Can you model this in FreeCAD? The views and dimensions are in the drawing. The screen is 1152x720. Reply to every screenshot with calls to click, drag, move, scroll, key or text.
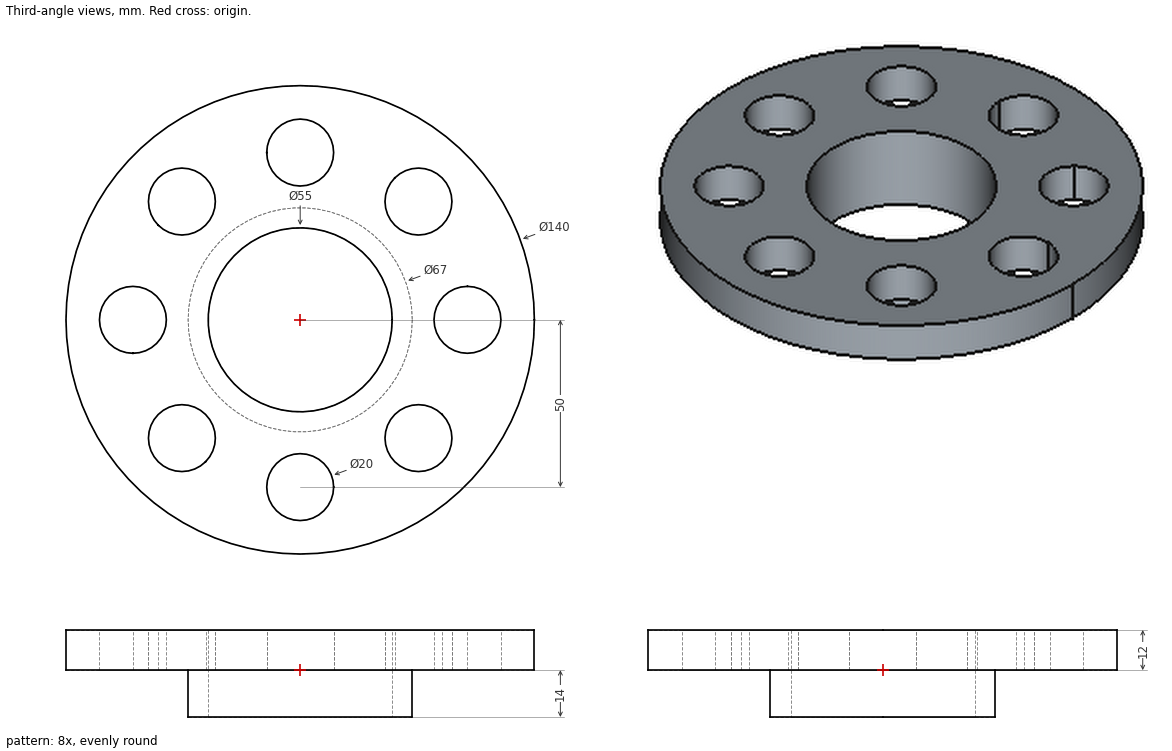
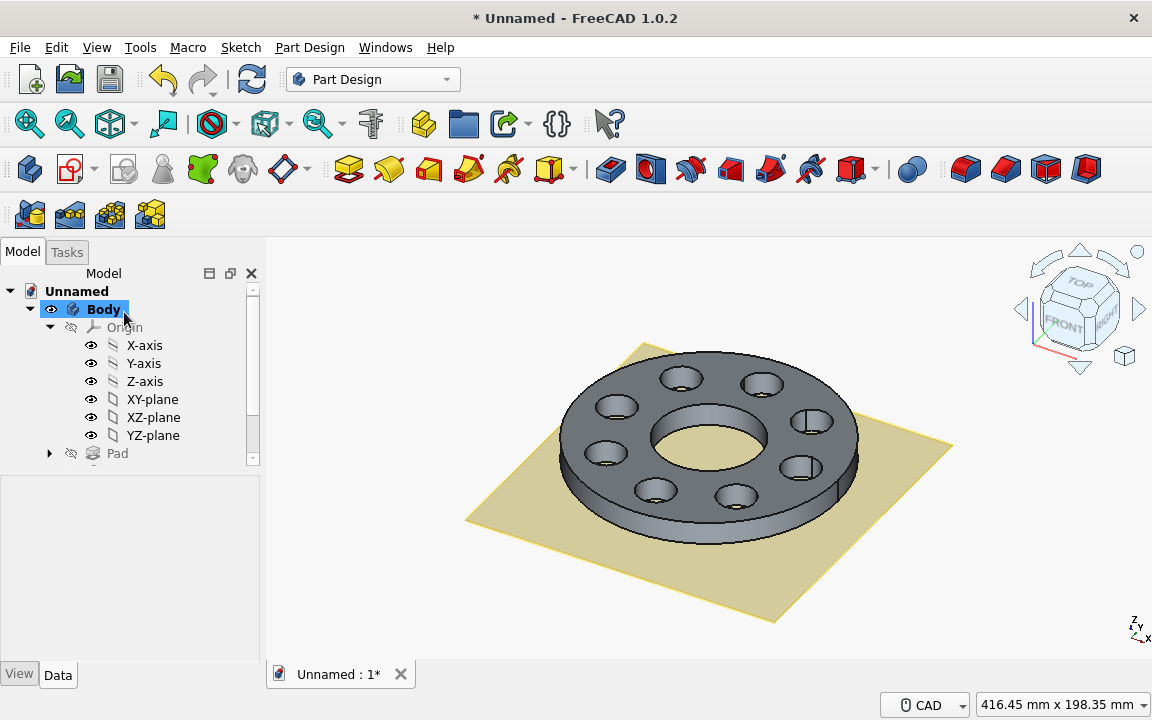
scroll(100, 377, down, 3)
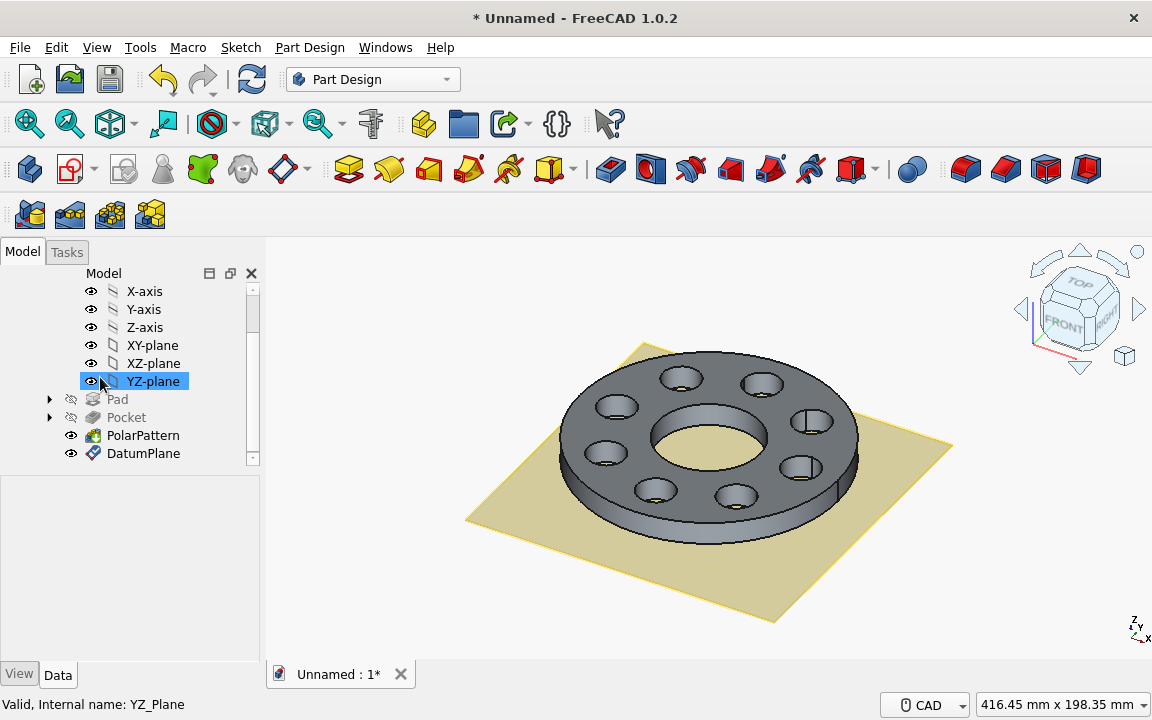
click(116, 453)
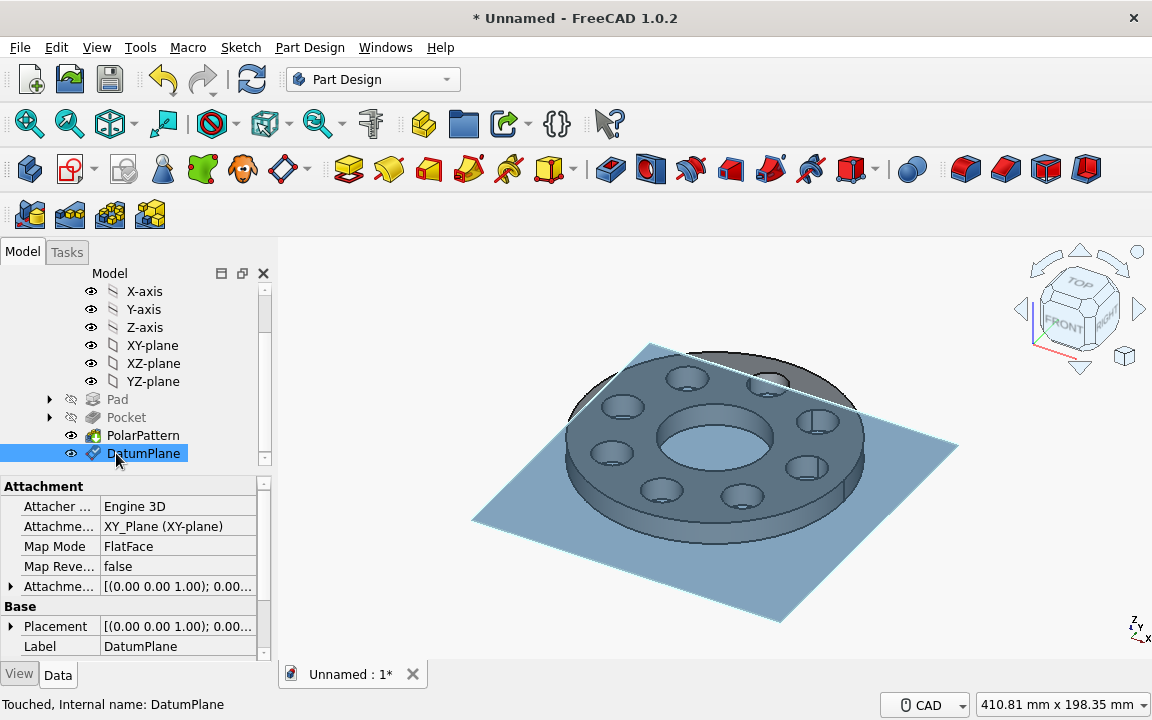
click(70, 170)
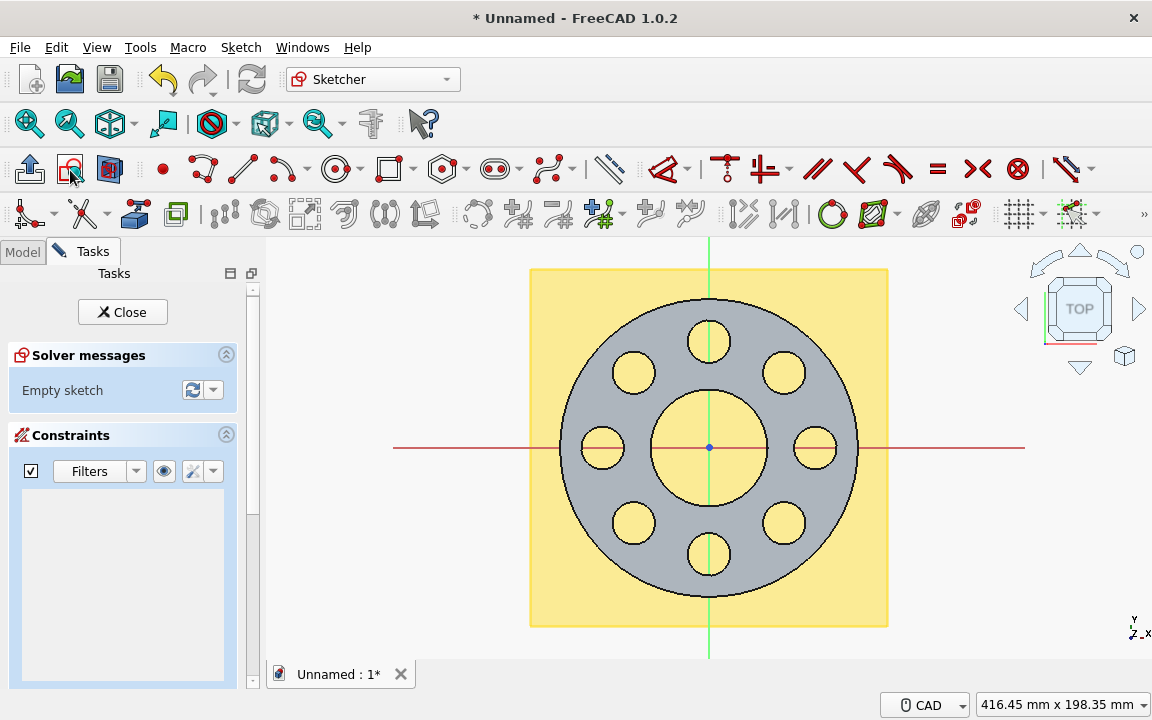
key(q)
key(s)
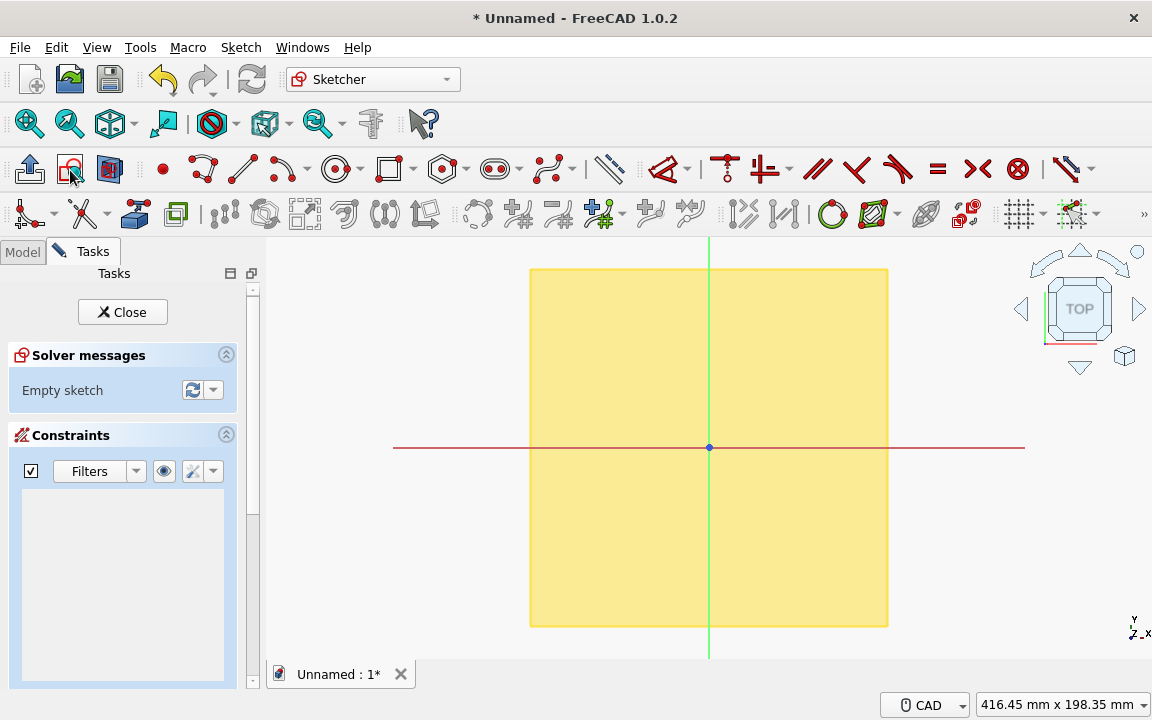
scroll(792, 448, up, 3)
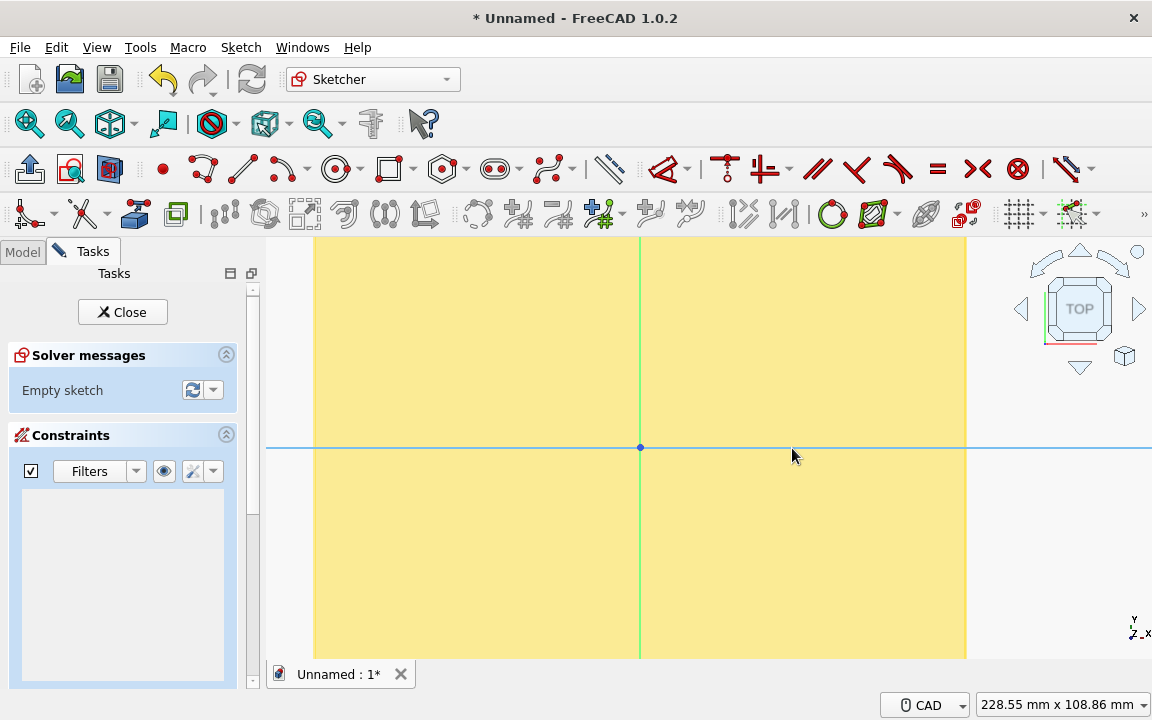
key(g)
key(c)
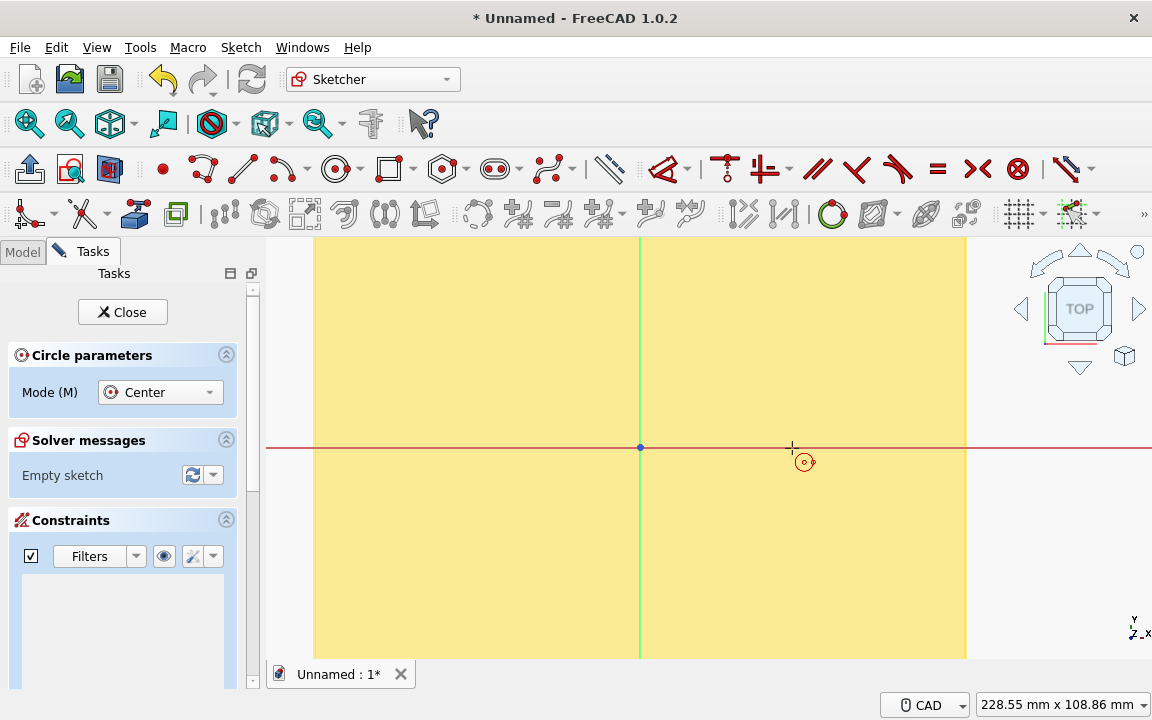
click(640, 448)
move(732, 356)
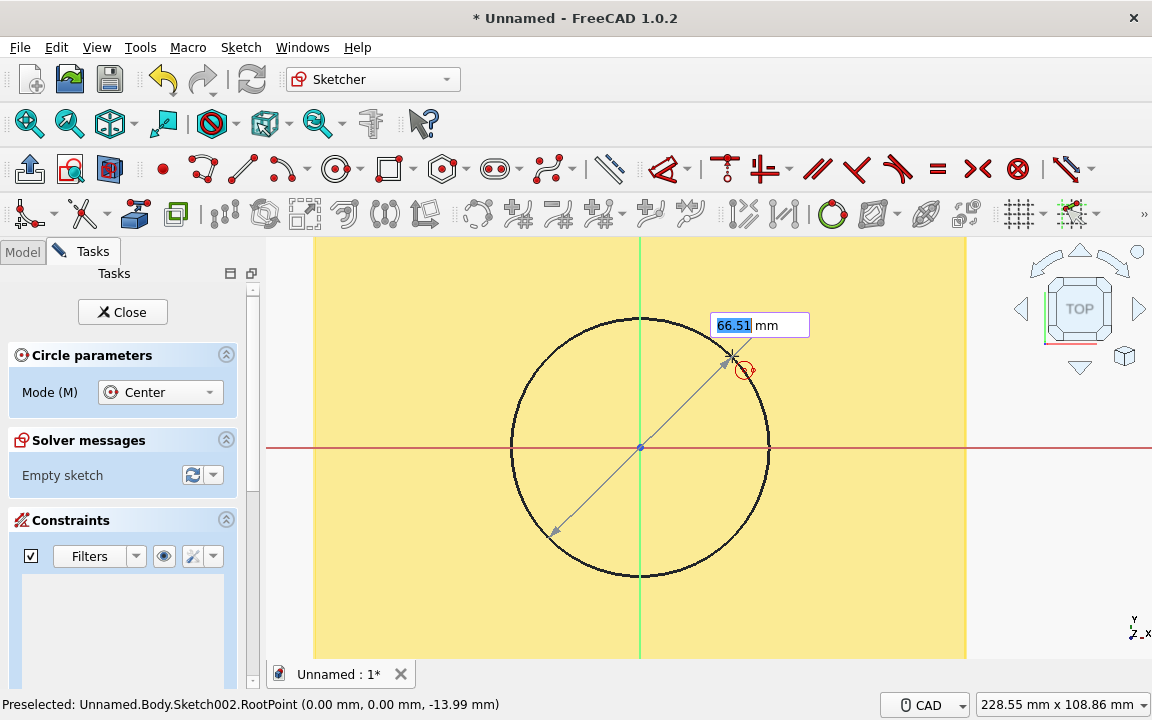
text(67)
key(Return)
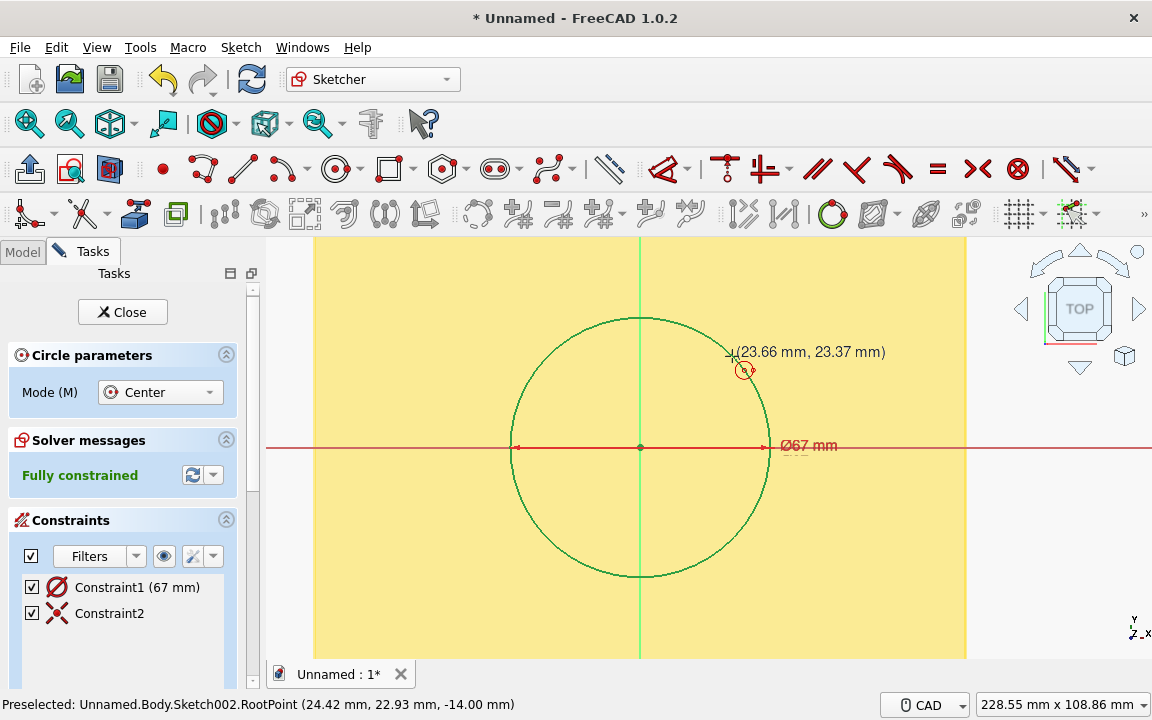
click(640, 448)
move(716, 372)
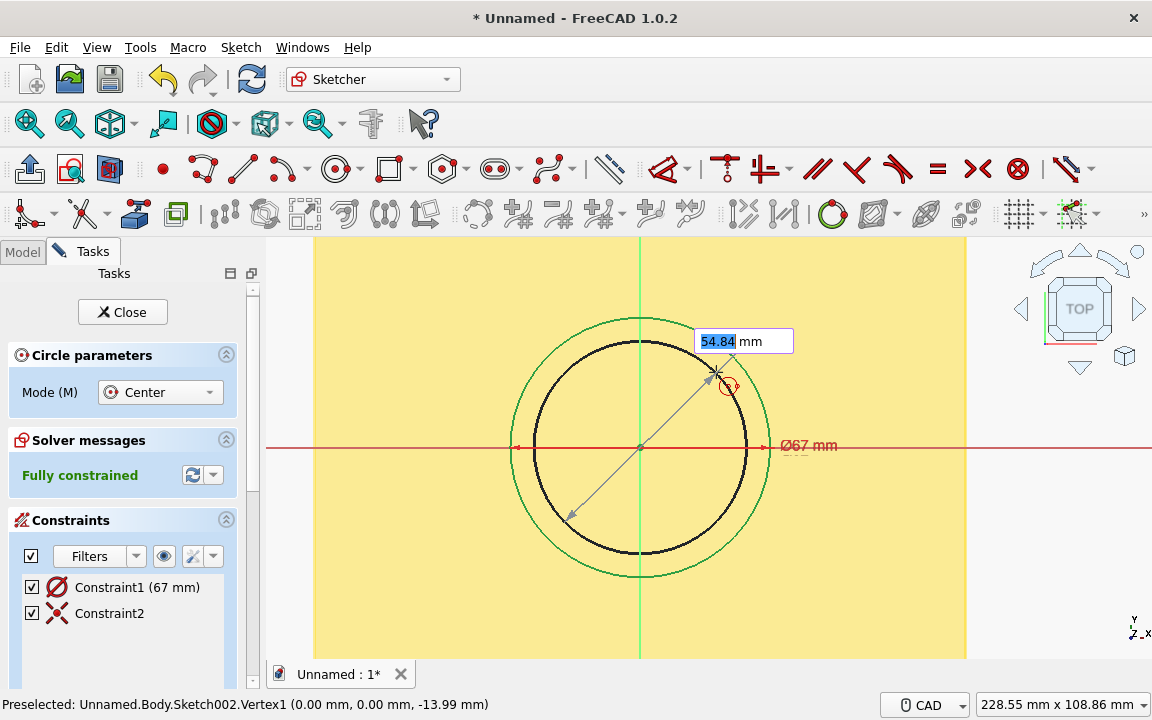
text(55)
key(Return)
key(Escape)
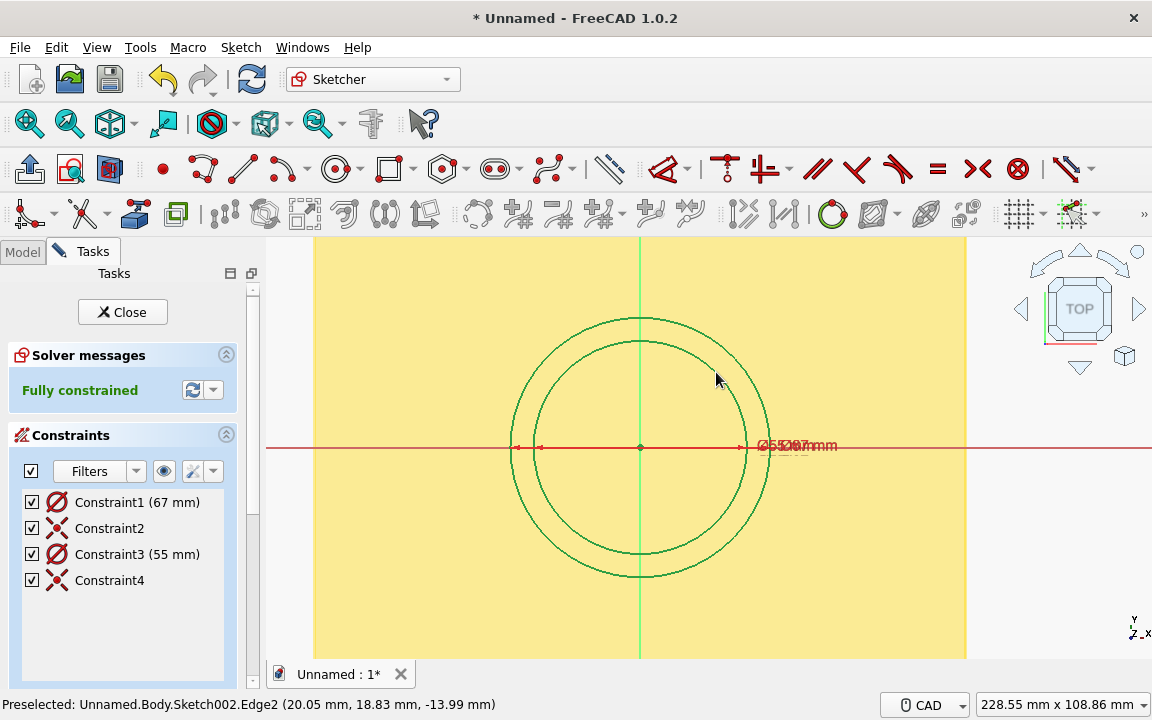
click(123, 312)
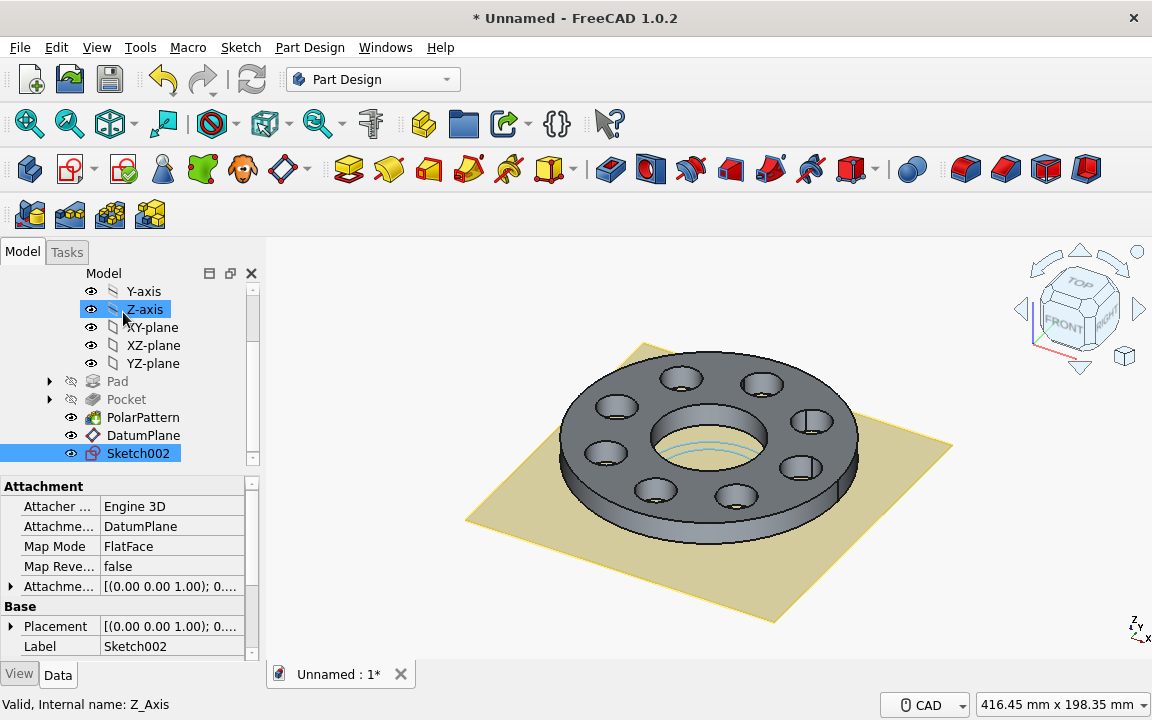
click(350, 170)